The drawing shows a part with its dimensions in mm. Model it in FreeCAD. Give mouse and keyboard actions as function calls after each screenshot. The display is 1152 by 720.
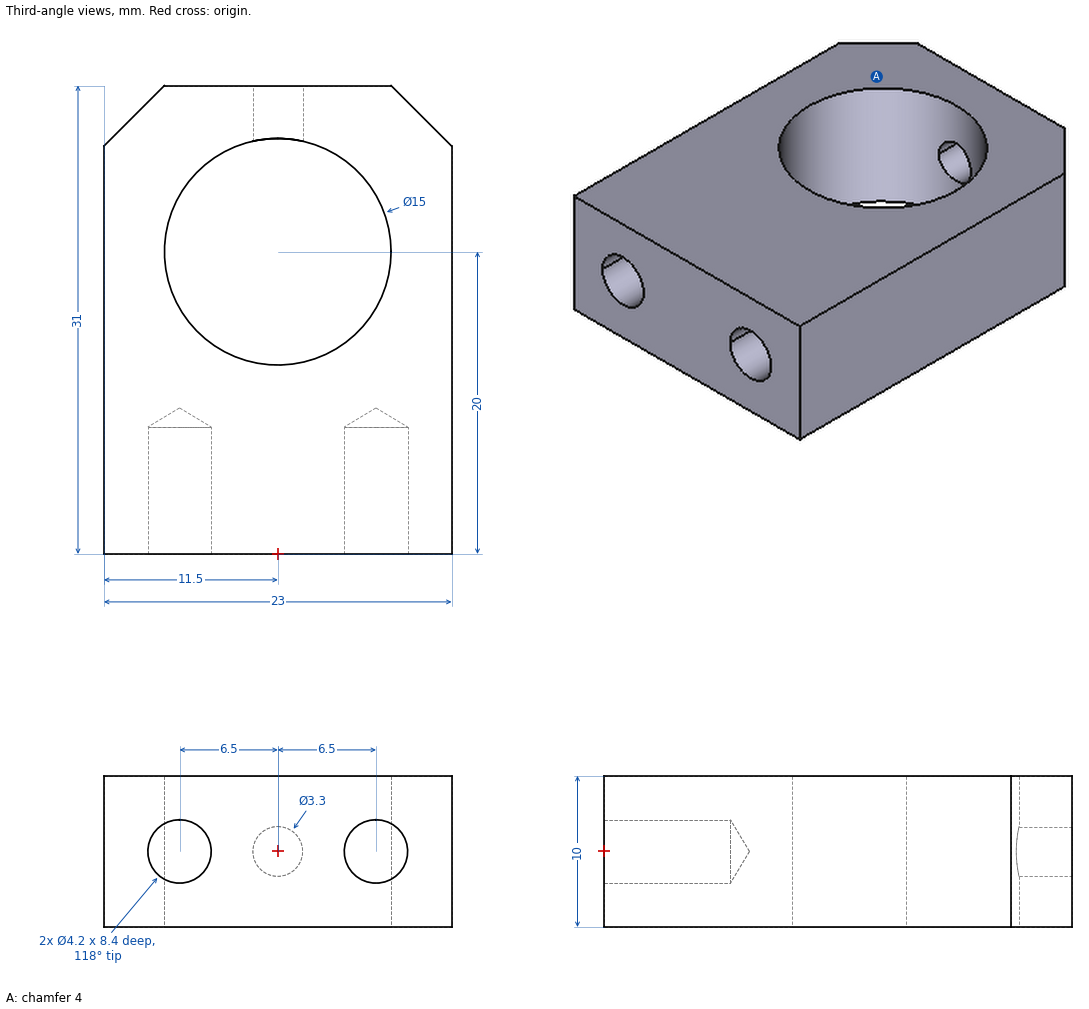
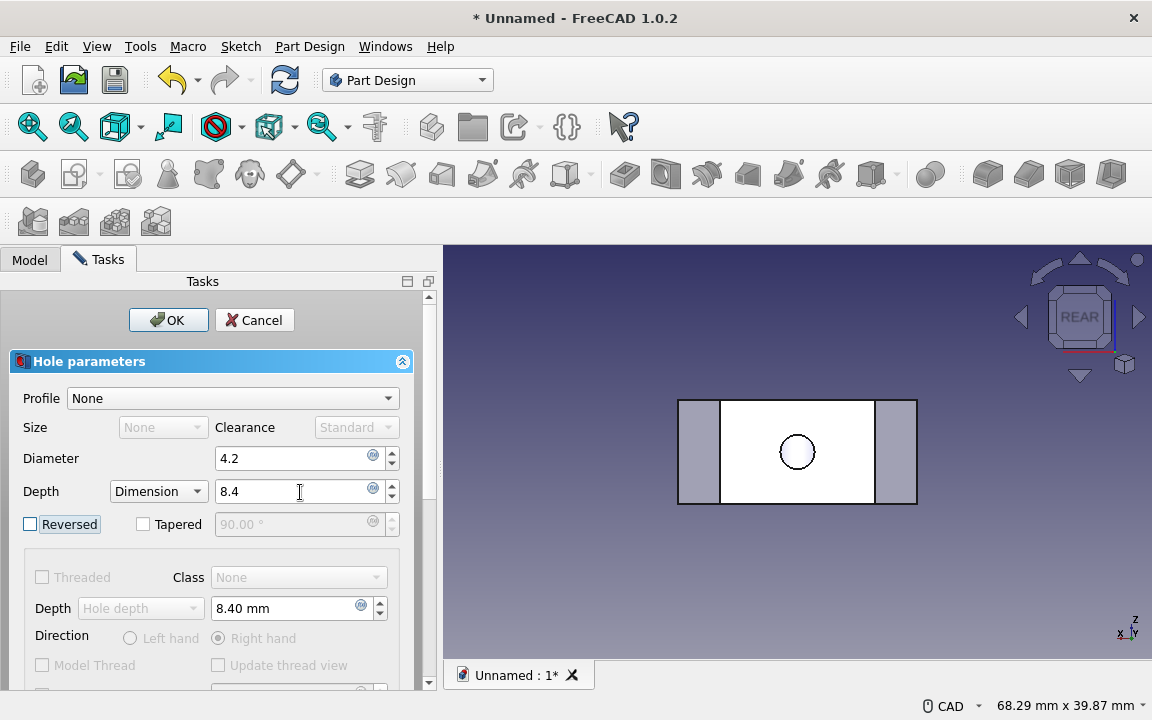
click(169, 320)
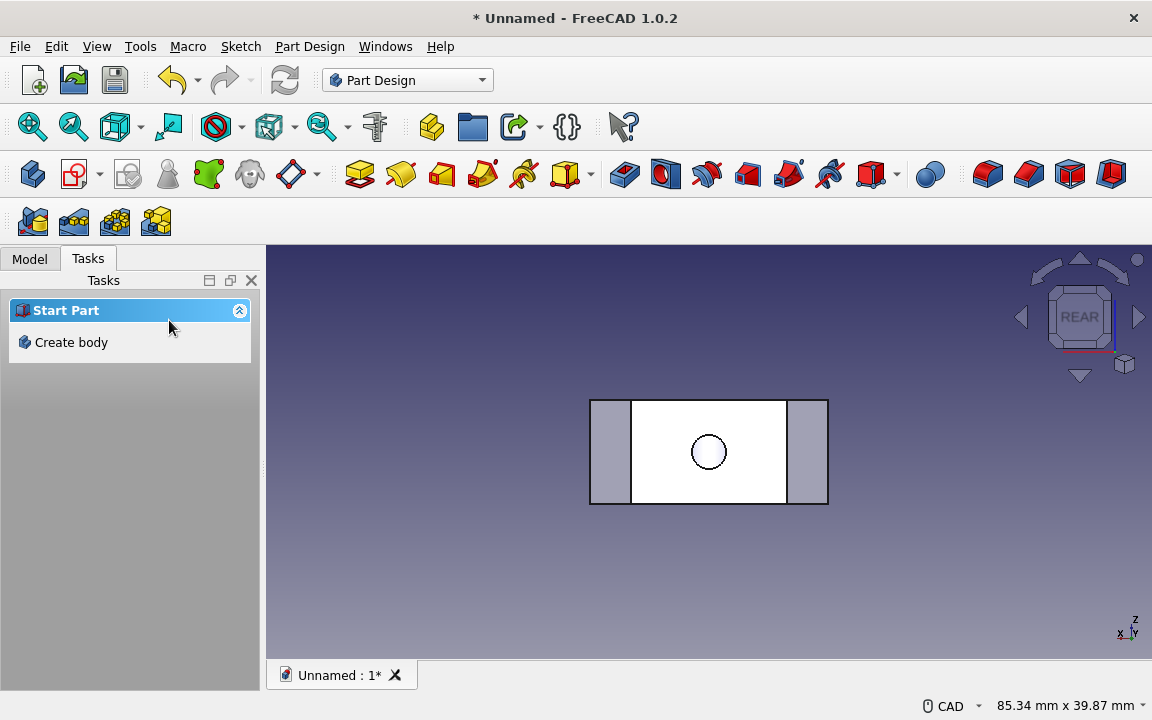
key(0)